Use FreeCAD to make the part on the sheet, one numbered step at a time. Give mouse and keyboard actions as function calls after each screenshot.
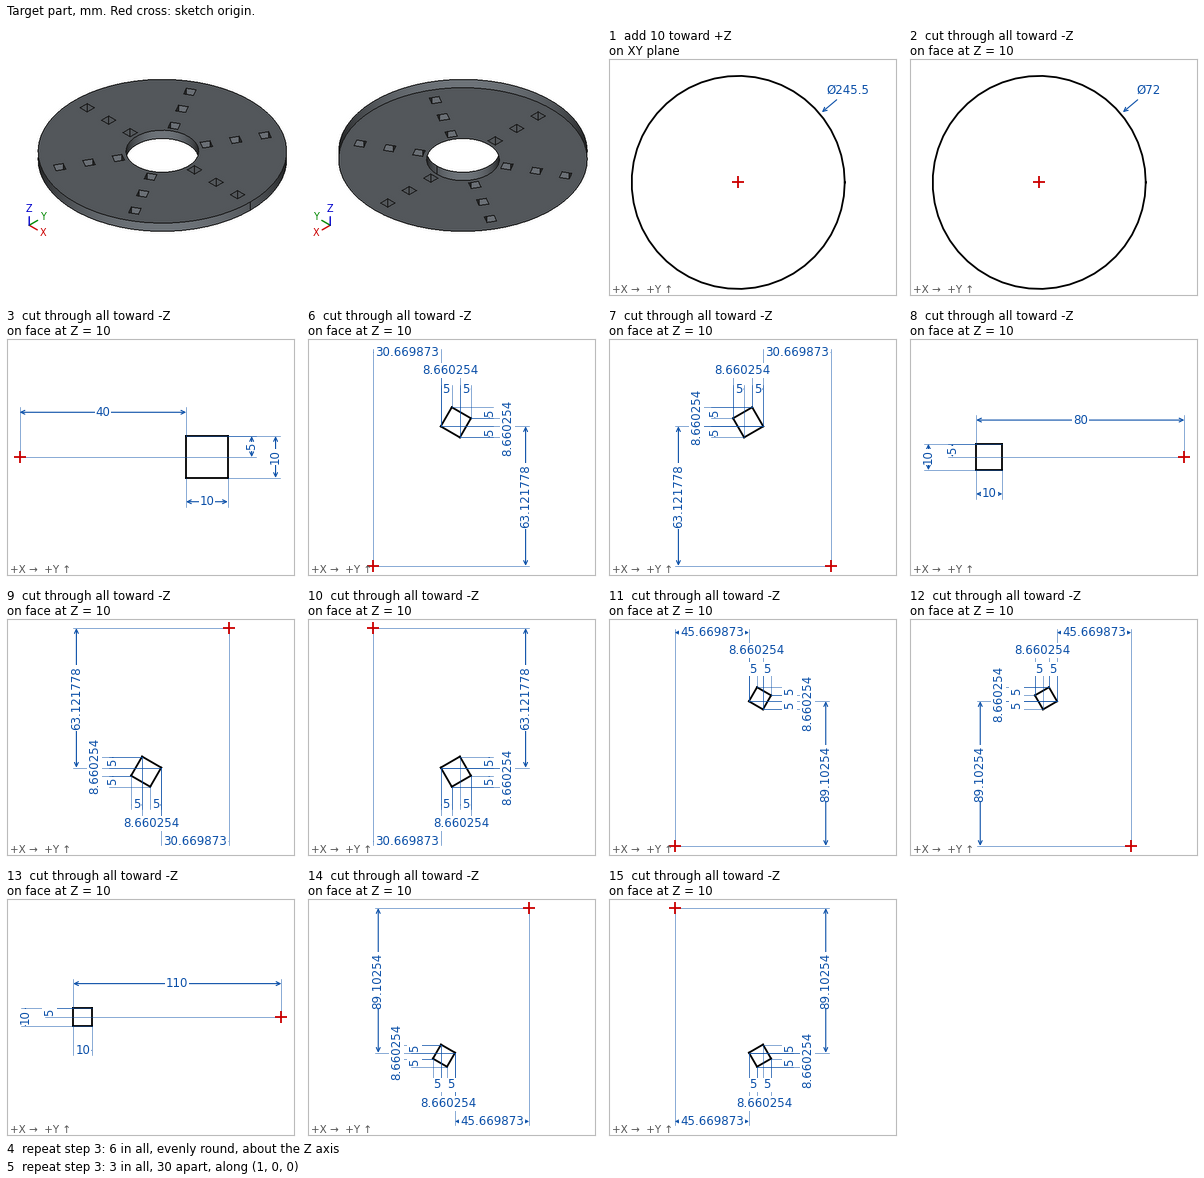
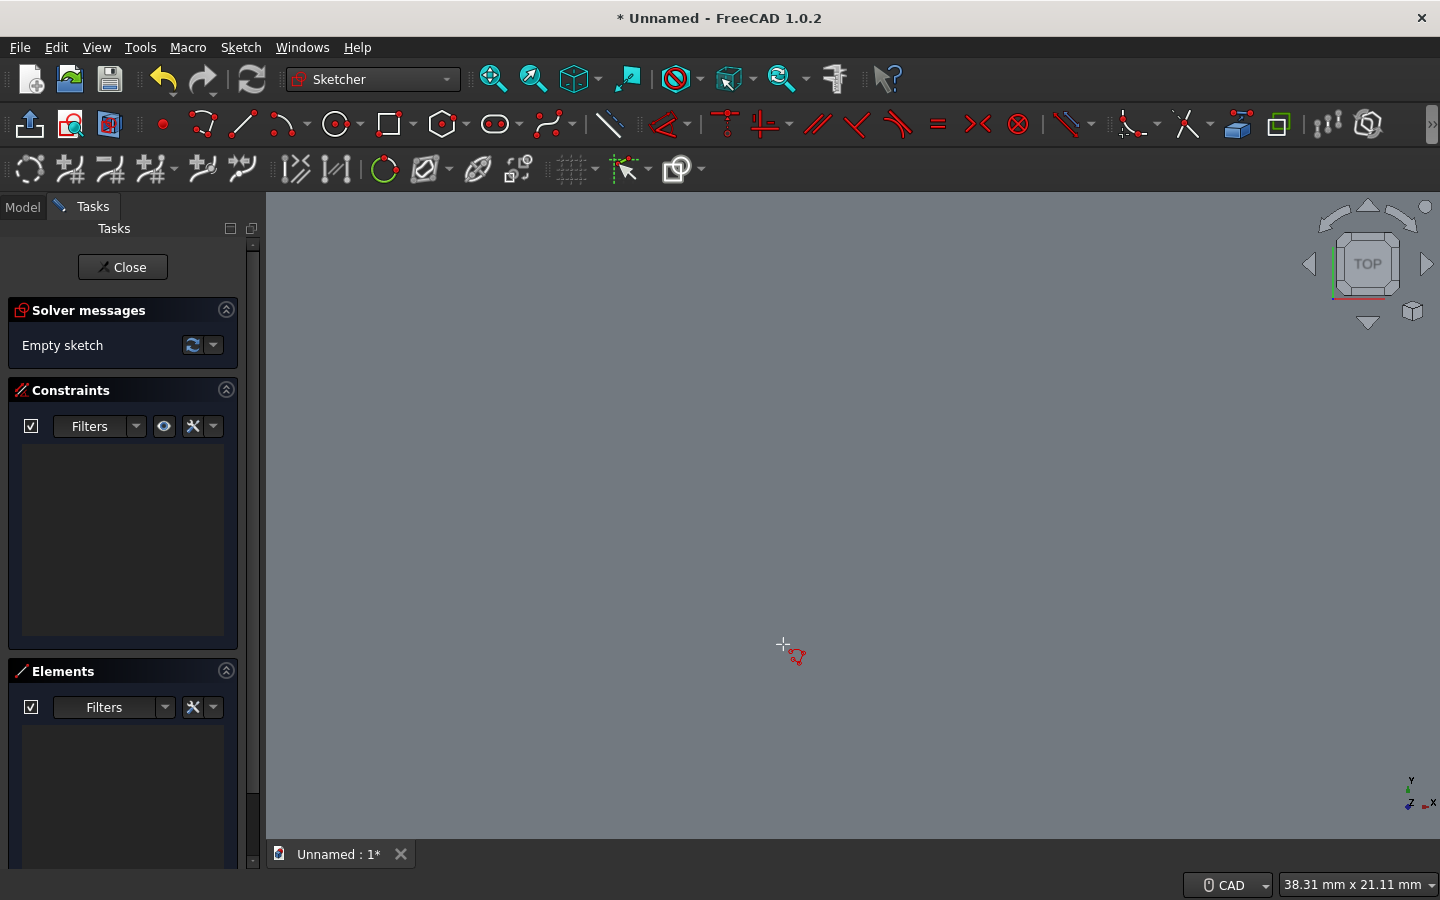
click(985, 455)
click(719, 301)
click(566, 567)
click(832, 720)
click(985, 456)
key(Escape)
key(Escape)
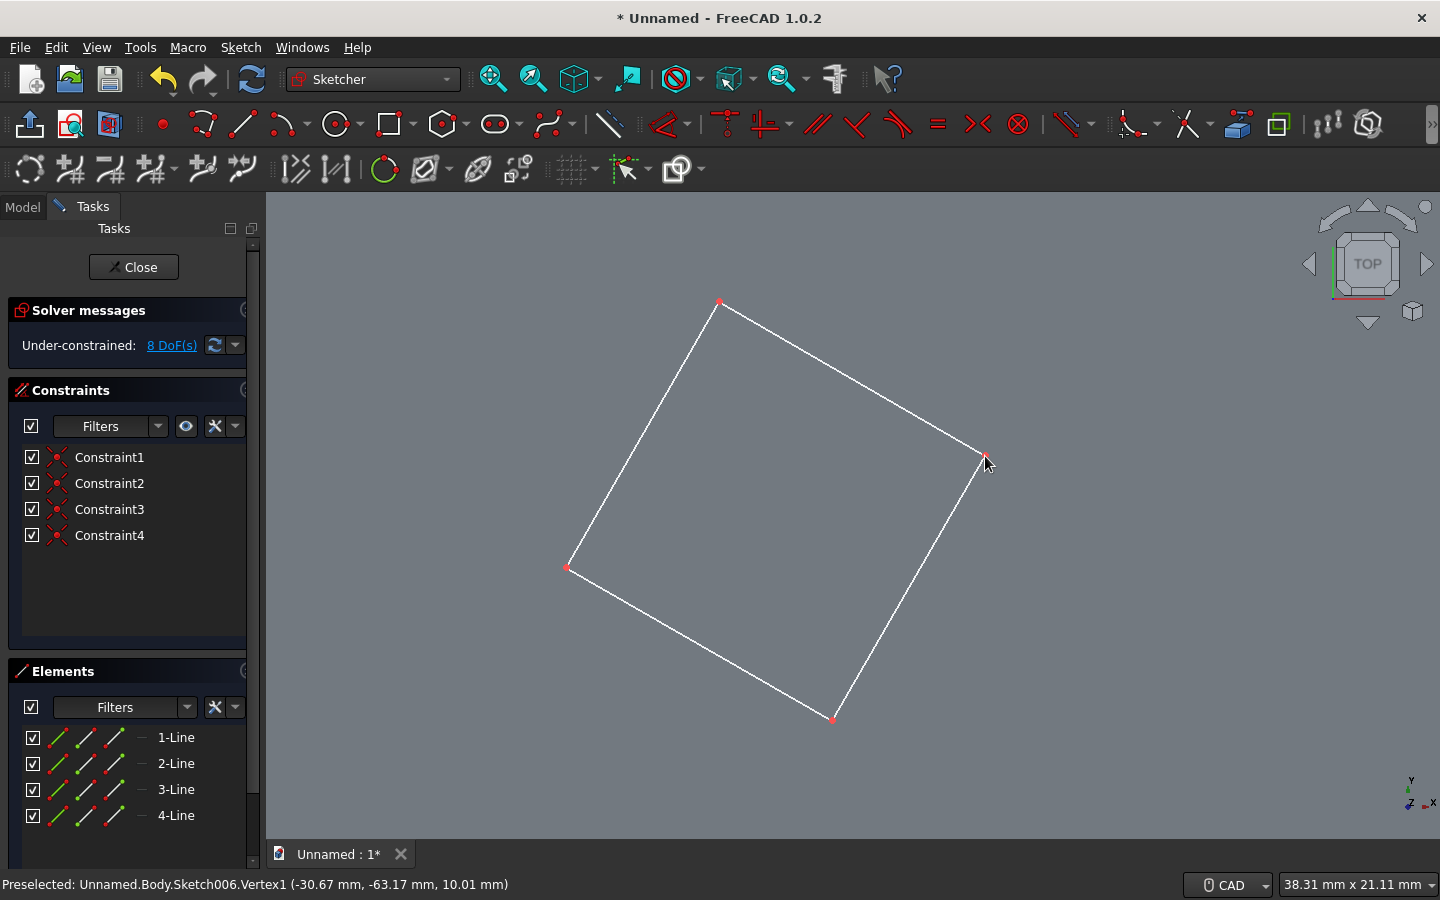
key(d)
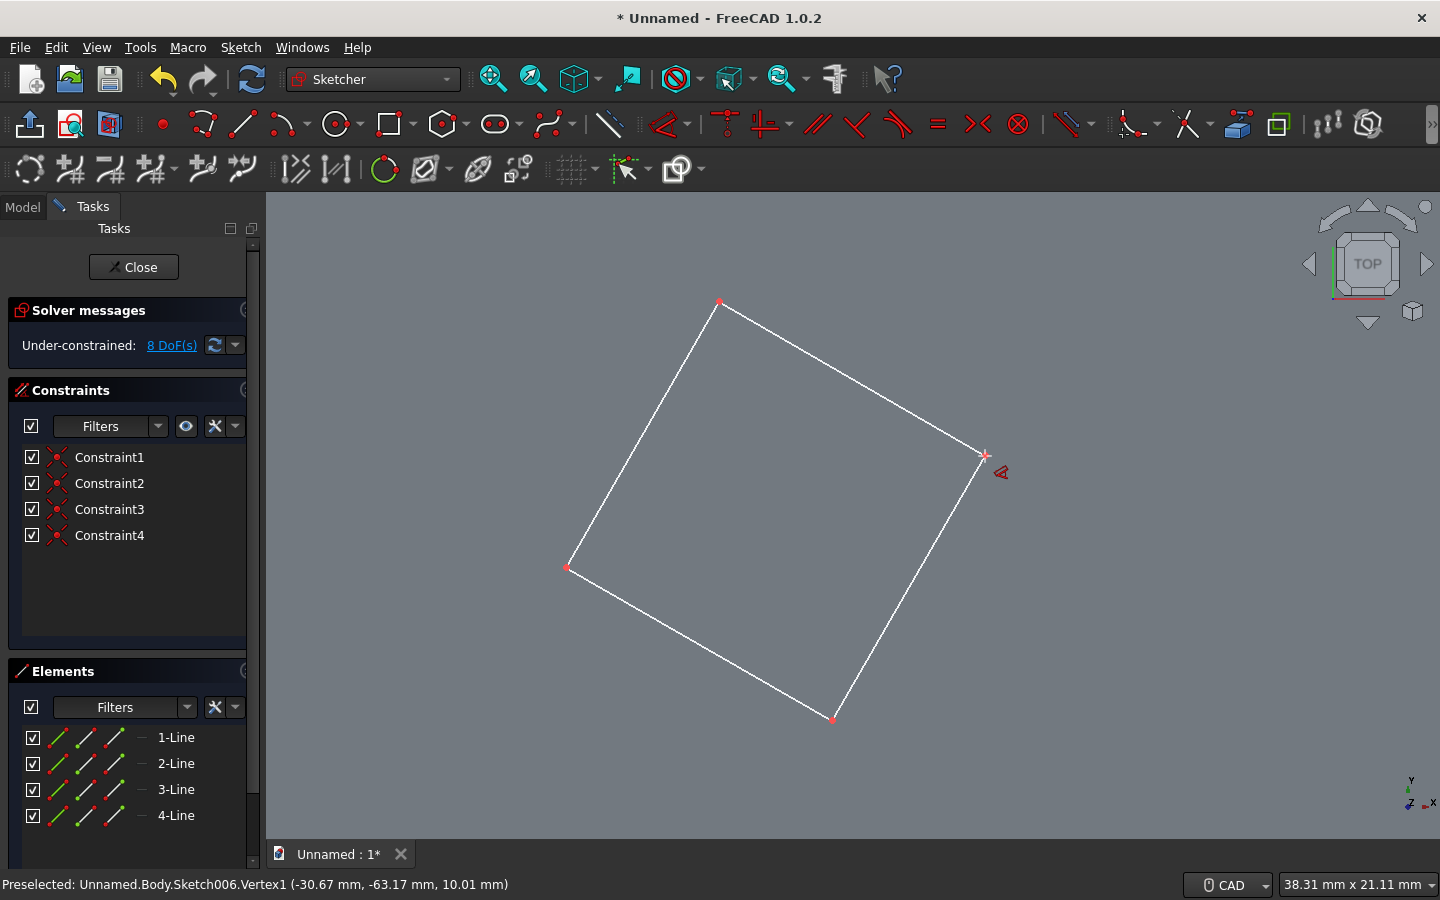
click(905, 410)
click(1019, 379)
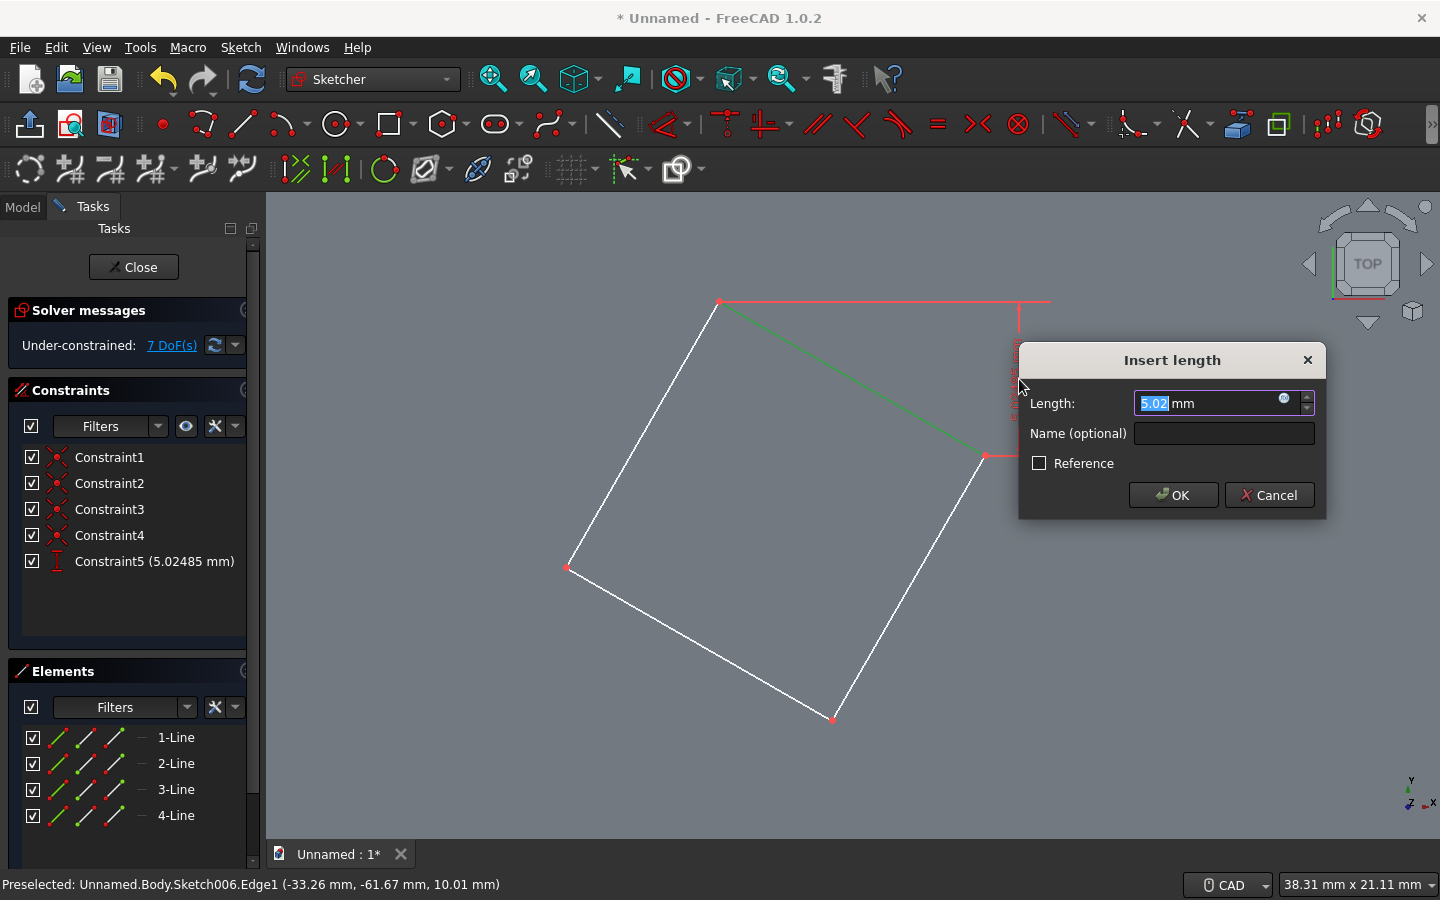
text(5)
key(Return)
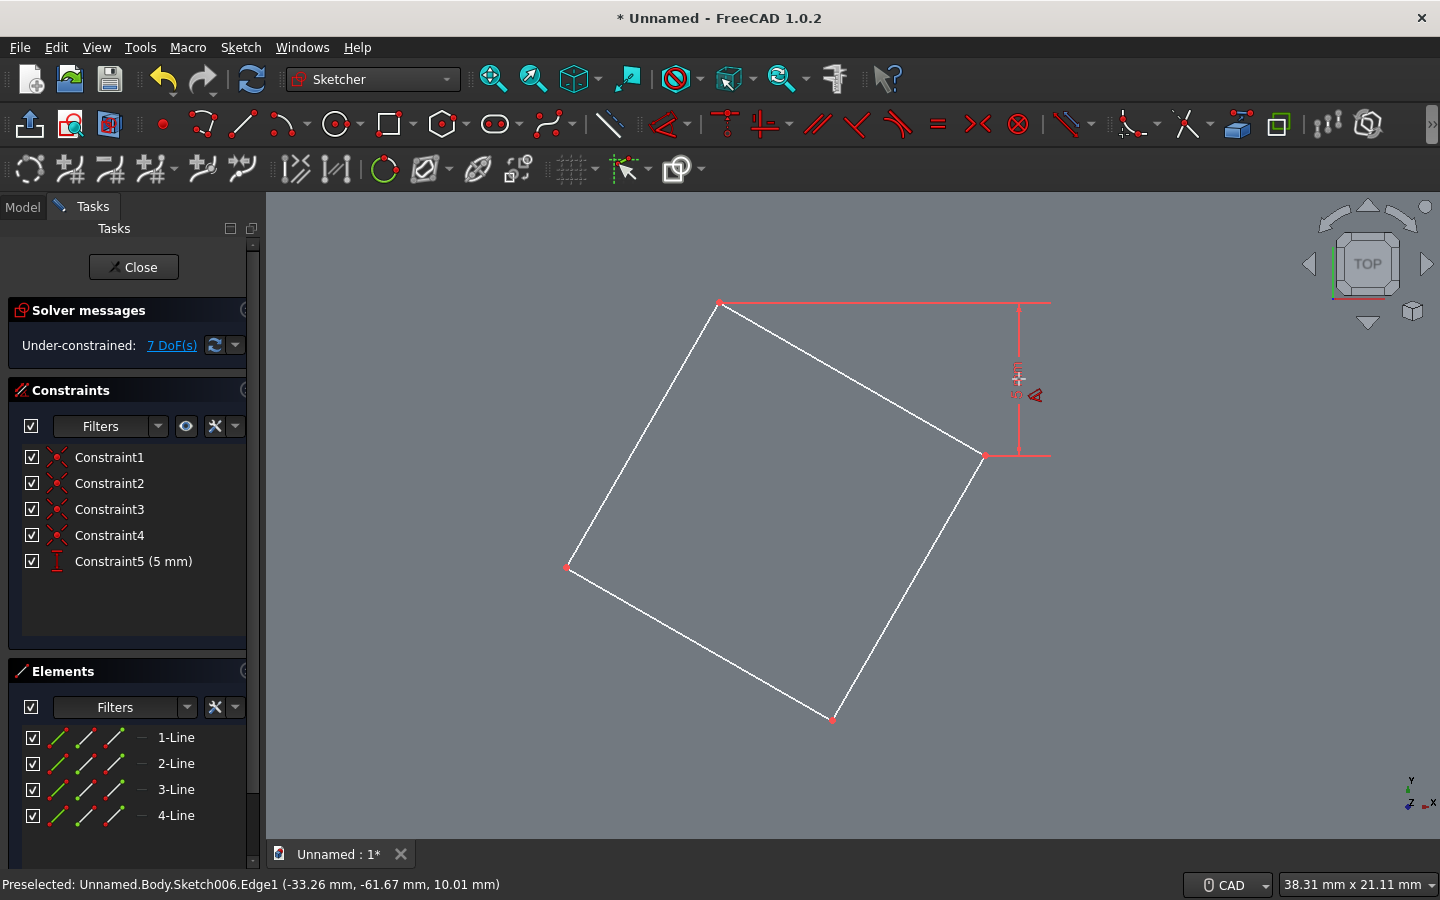
click(673, 382)
click(642, 269)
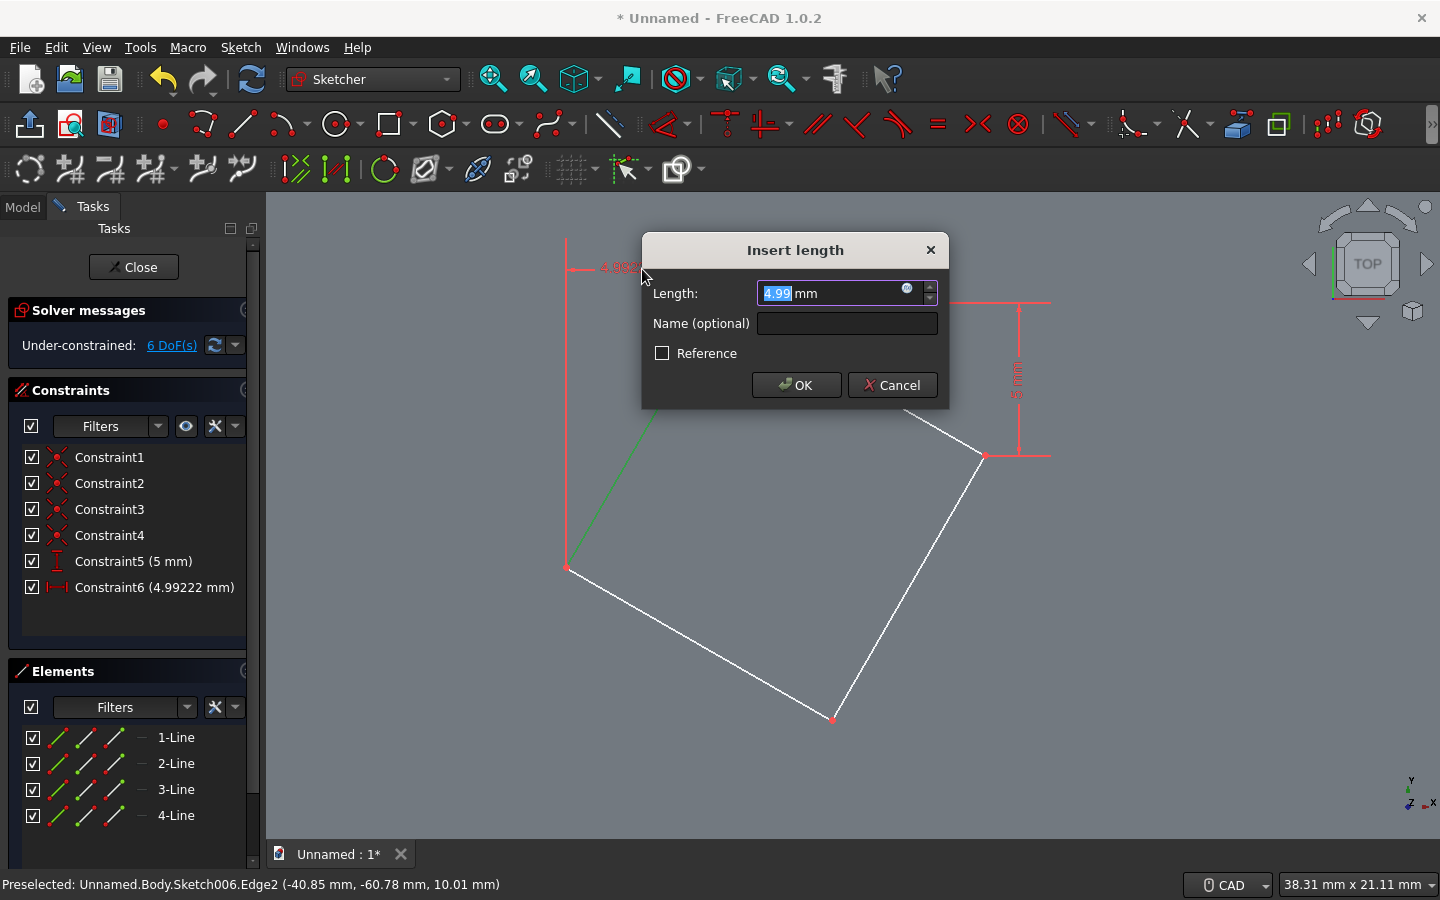
text(5)
key(Return)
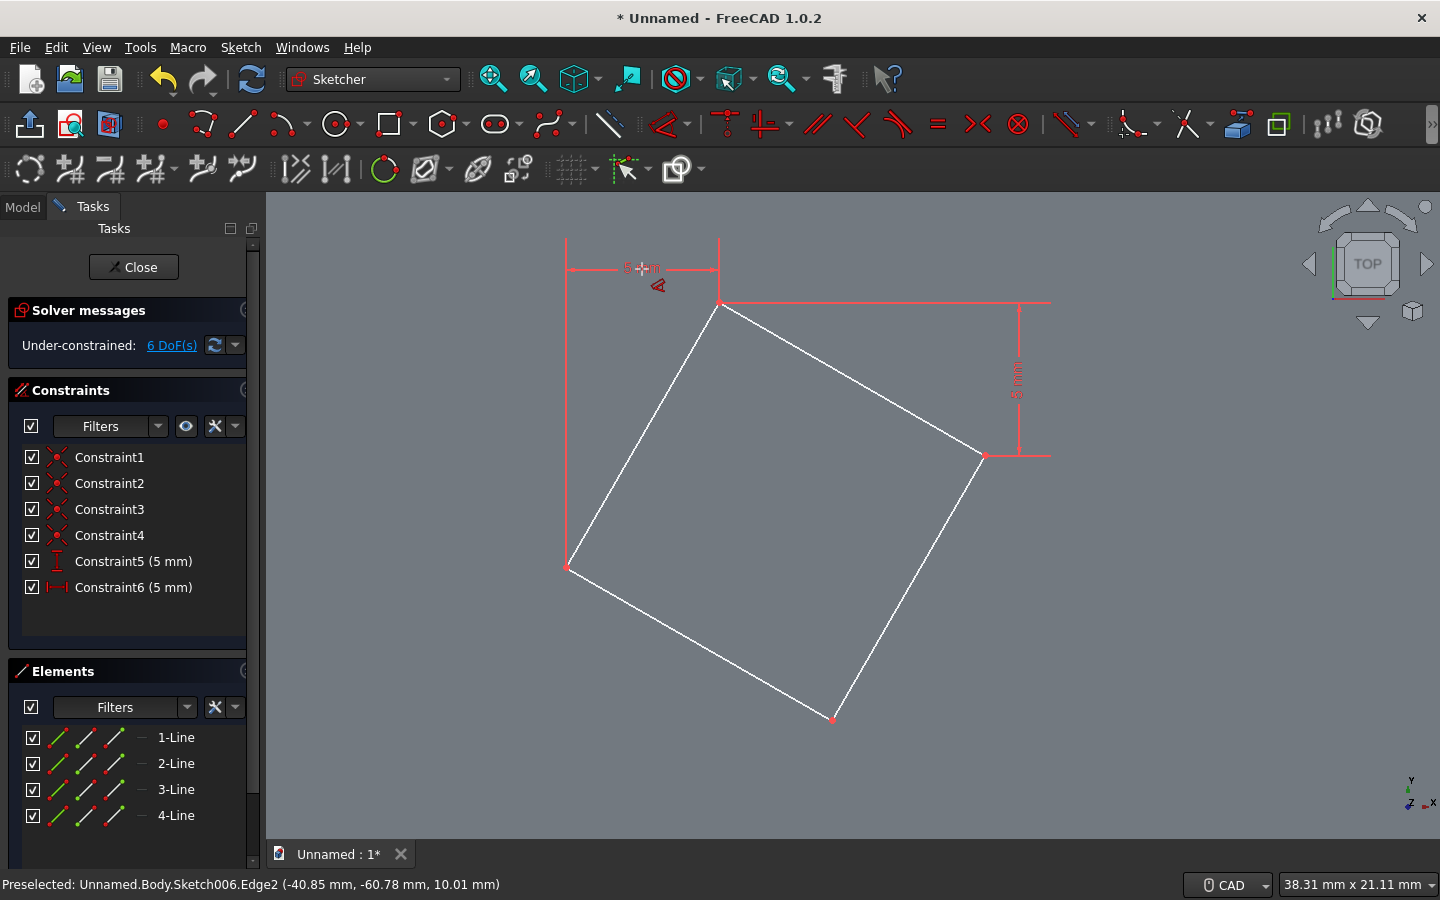
click(646, 614)
click(532, 644)